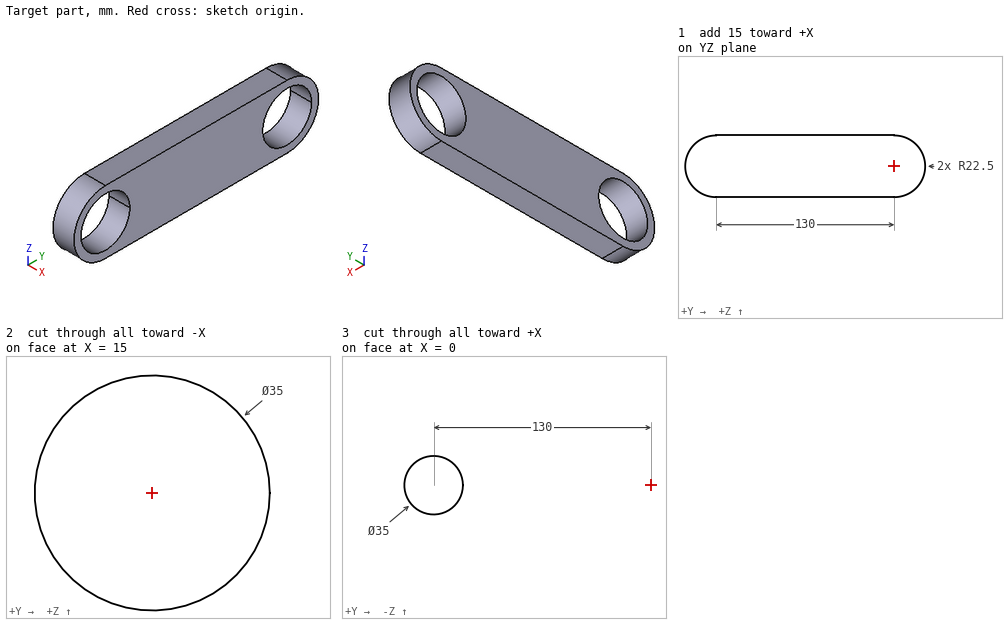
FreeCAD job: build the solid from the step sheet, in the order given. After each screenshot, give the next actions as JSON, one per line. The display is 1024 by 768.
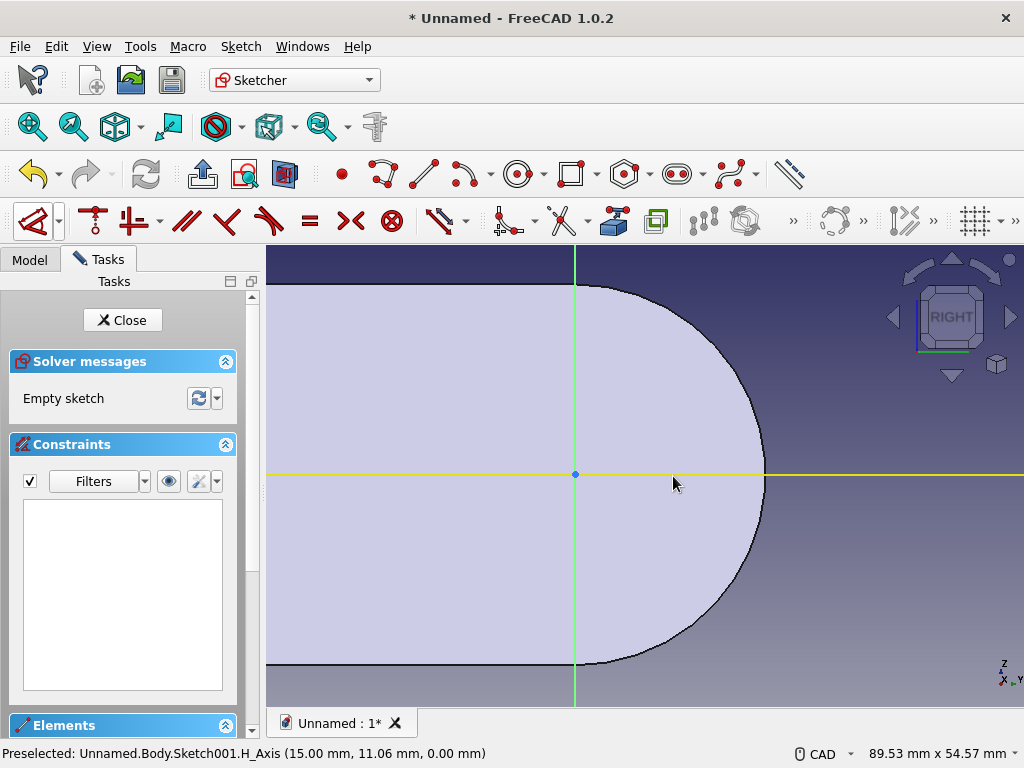
{"action": "left_click", "coordinate": [518, 174]}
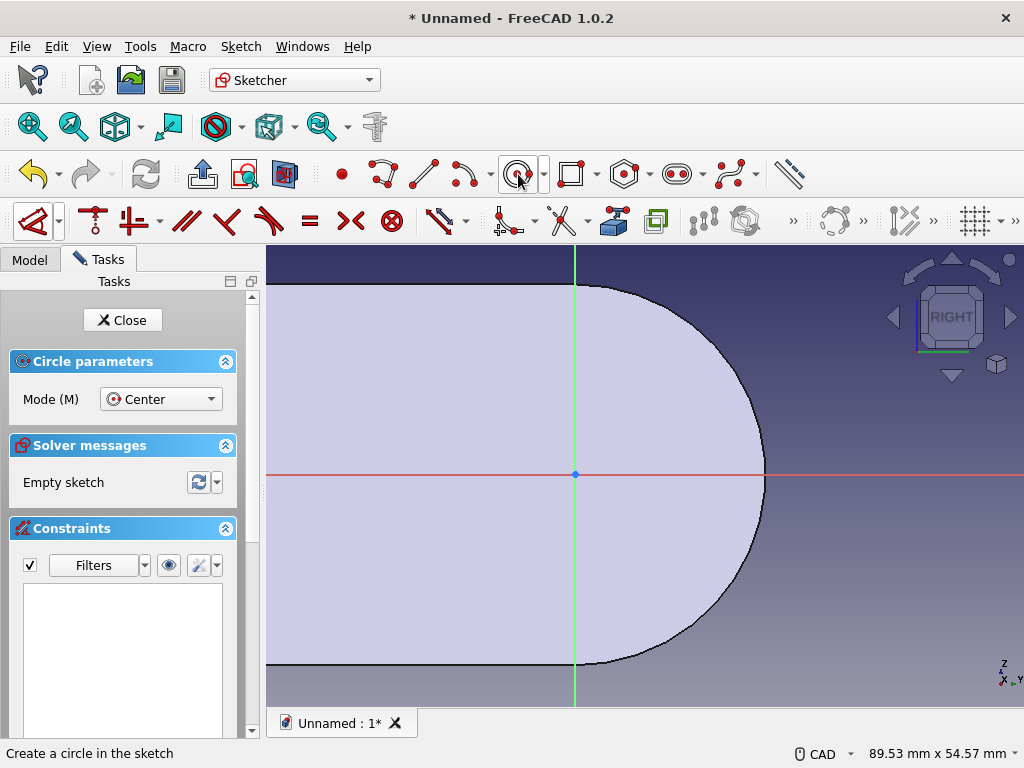
{"action": "left_click", "coordinate": [575, 475]}
{"action": "left_click", "coordinate": [680, 370]}
{"action": "key", "text": "Escape"}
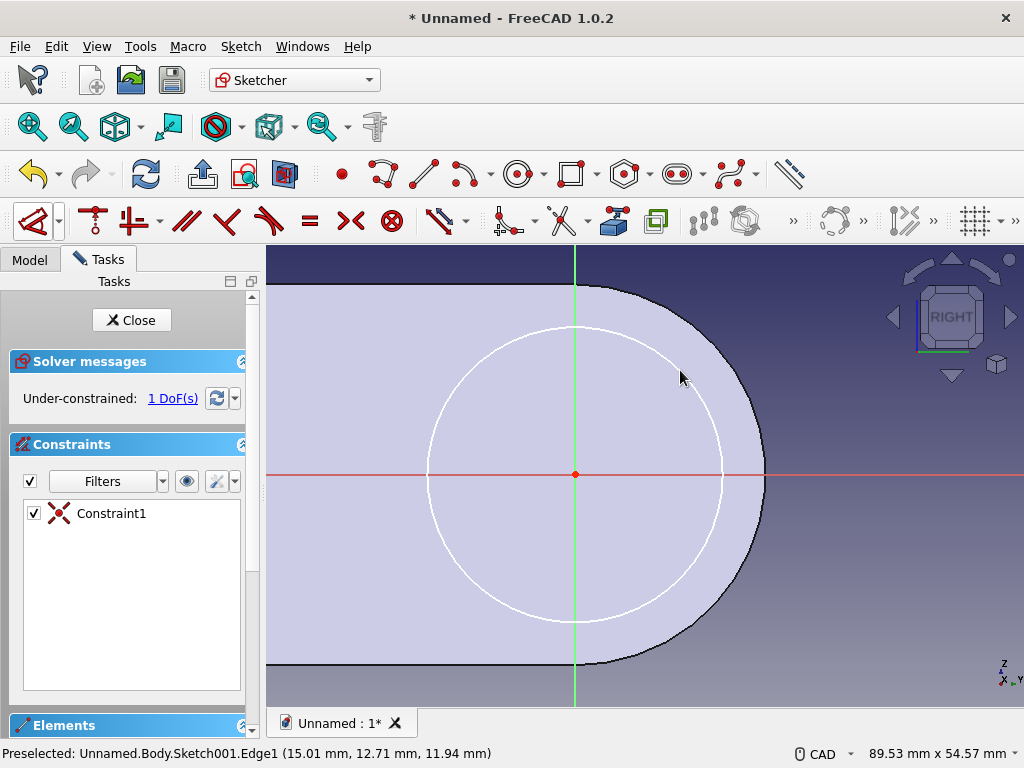
{"action": "left_click", "coordinate": [679, 370]}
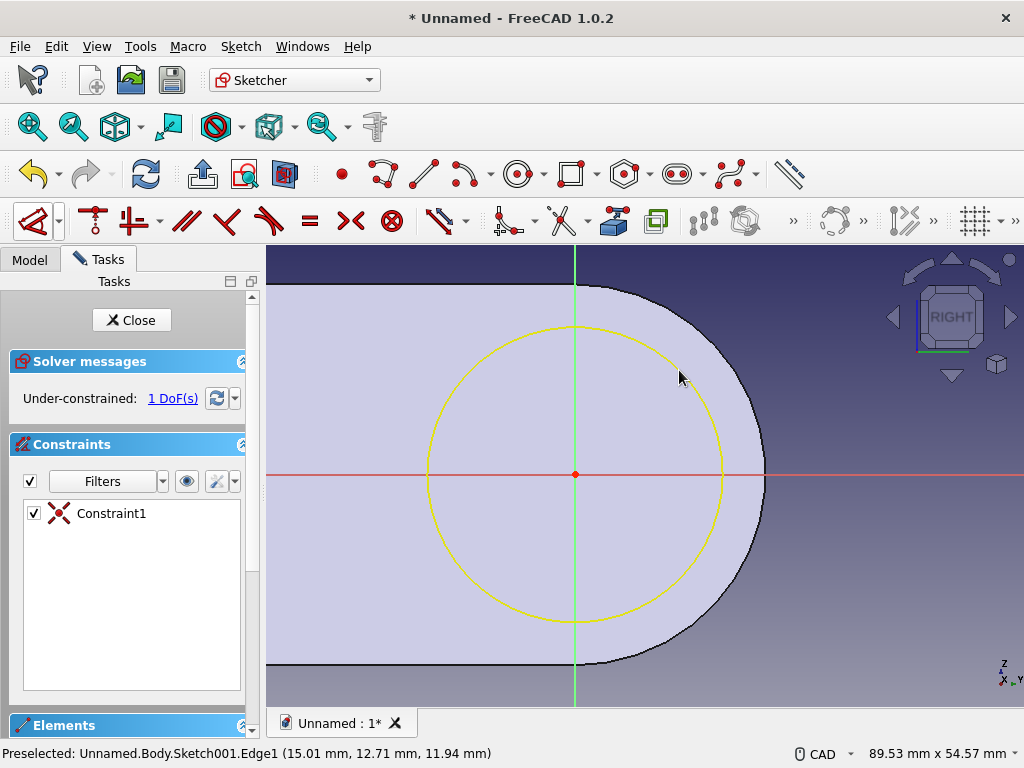
{"action": "left_click", "coordinate": [58, 222]}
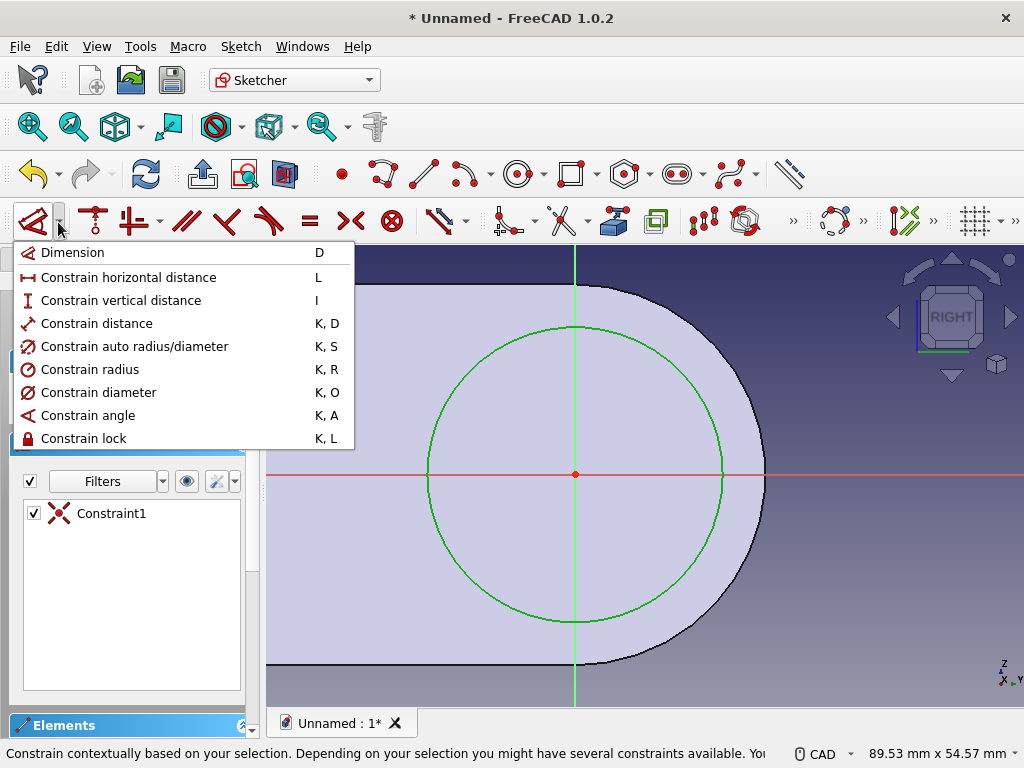
{"action": "left_click", "coordinate": [184, 392]}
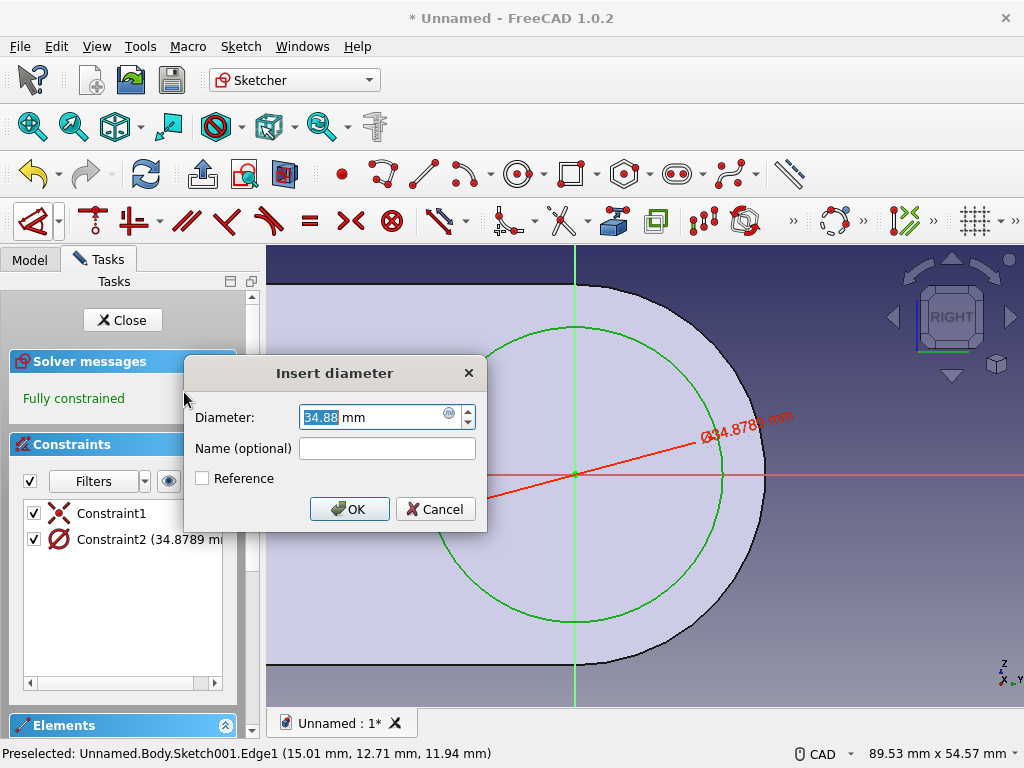
{"action": "type", "text": "35"}
{"action": "key", "text": "Return"}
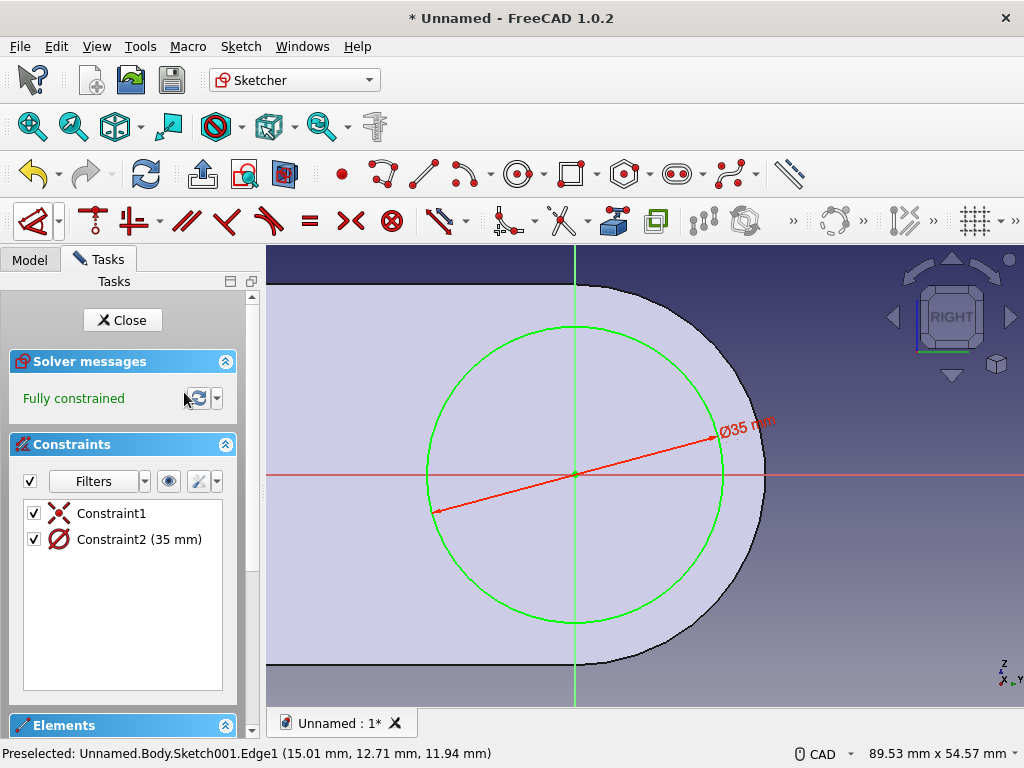
{"action": "left_click", "coordinate": [123, 320]}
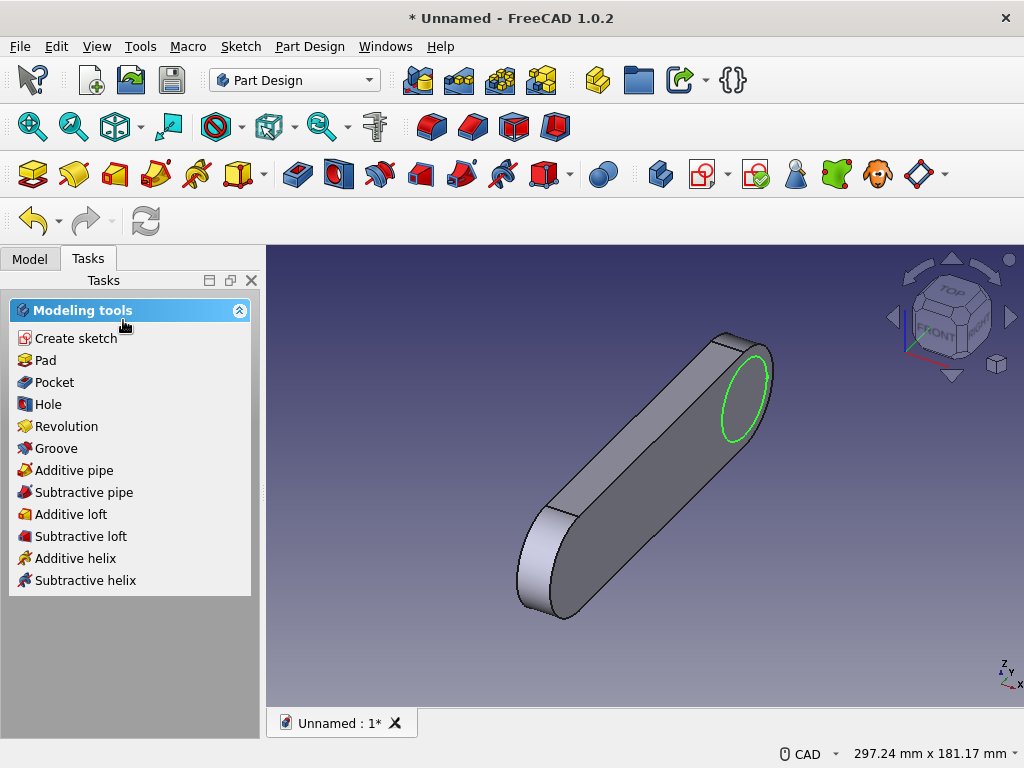
{"action": "left_click", "coordinate": [298, 174]}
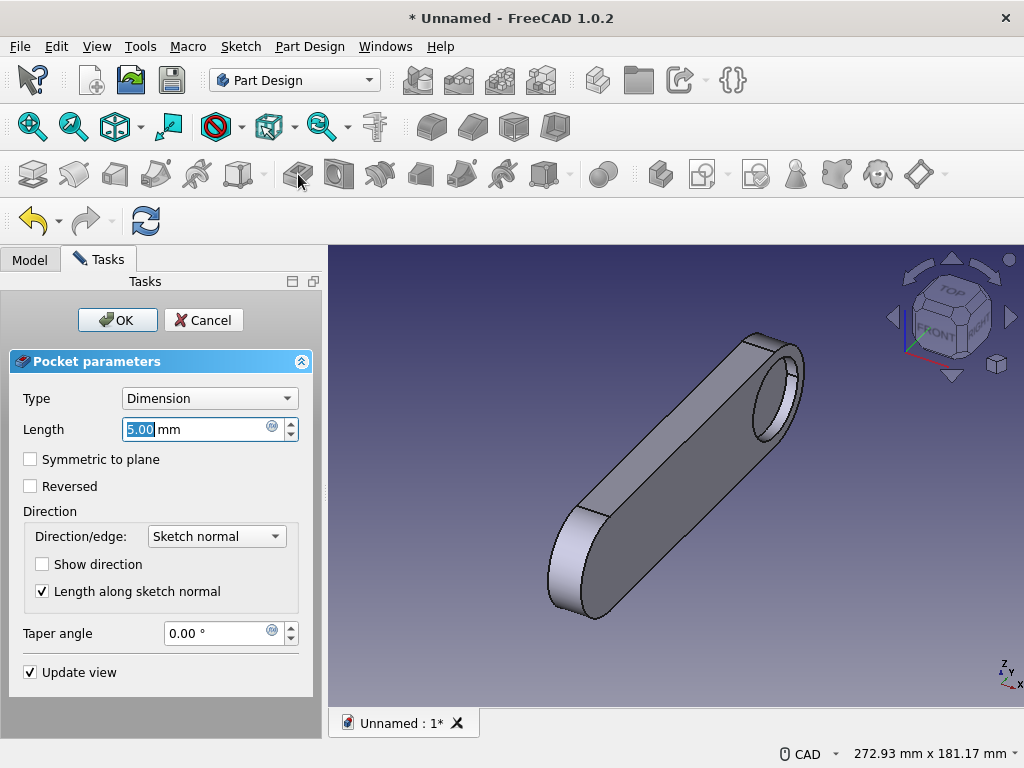
{"action": "left_click", "coordinate": [210, 398]}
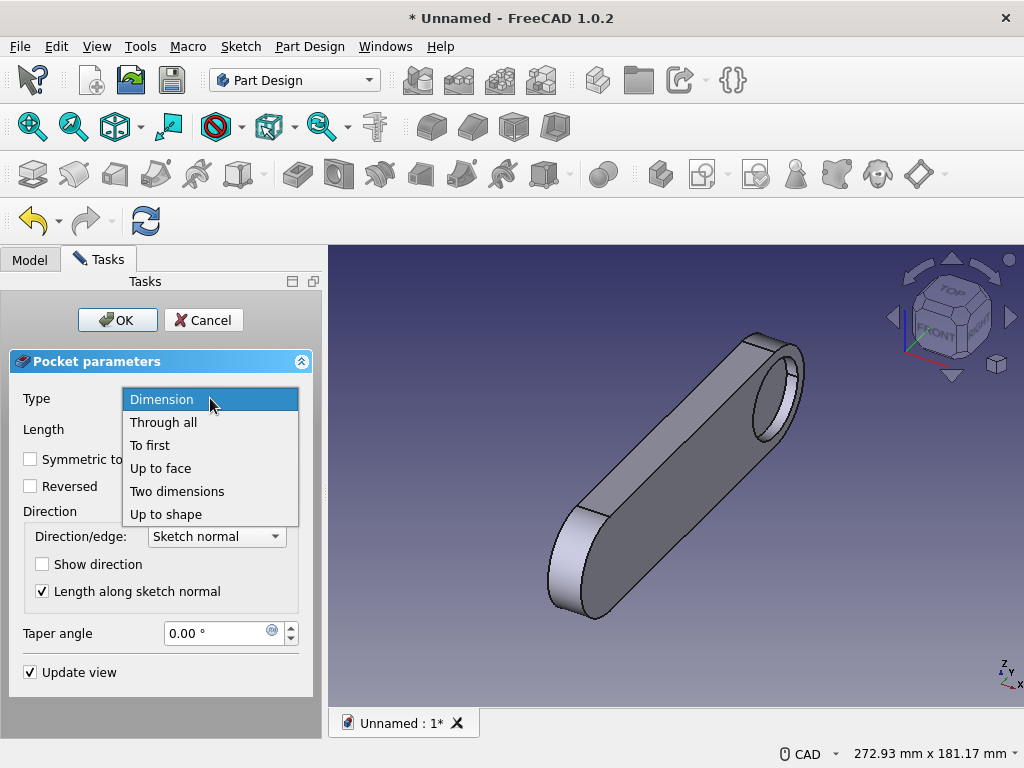
{"action": "left_click", "coordinate": [208, 422]}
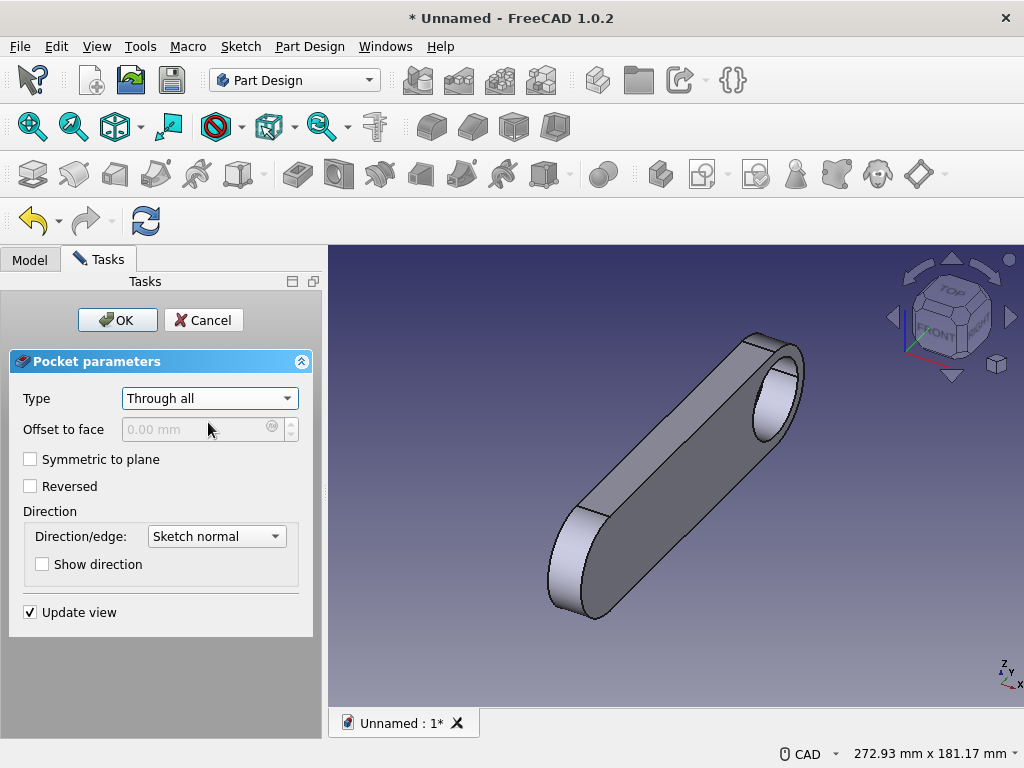
{"action": "left_click", "coordinate": [118, 320]}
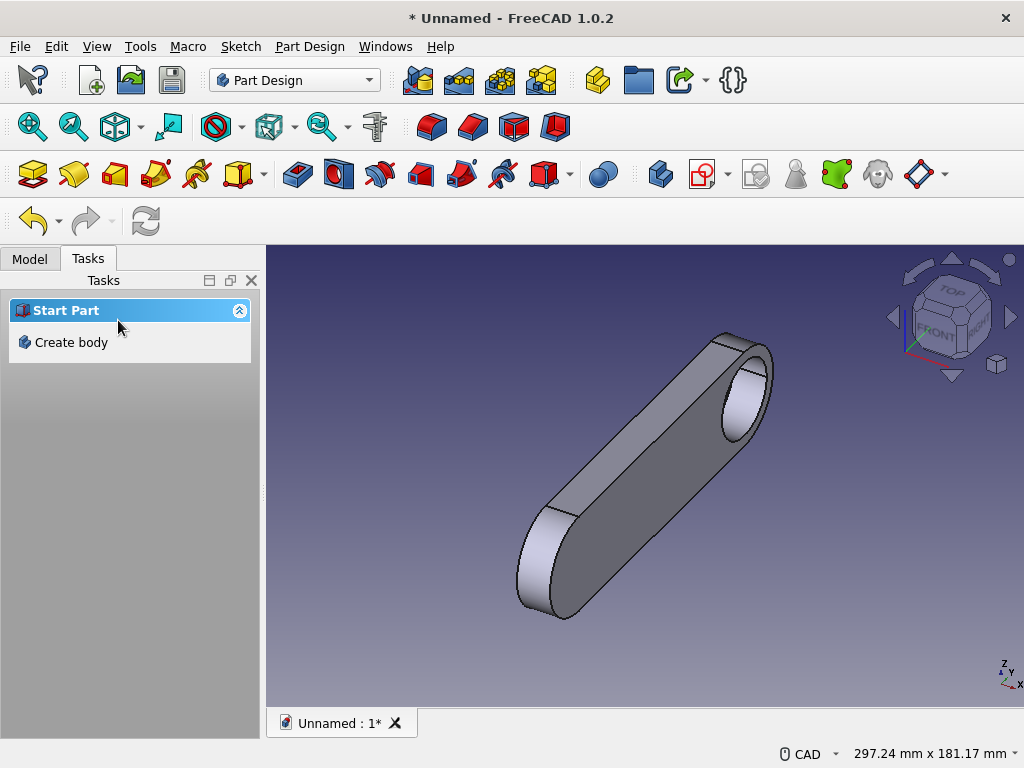
{"action": "key", "text": "6"}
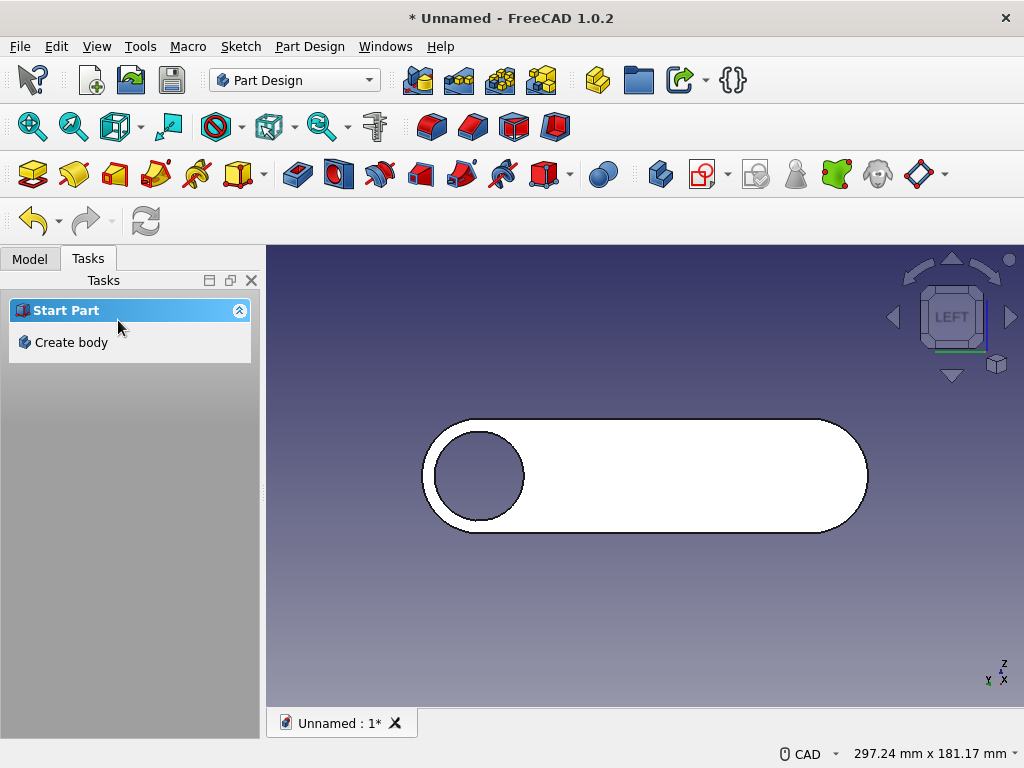
{"action": "left_click", "coordinate": [645, 475]}